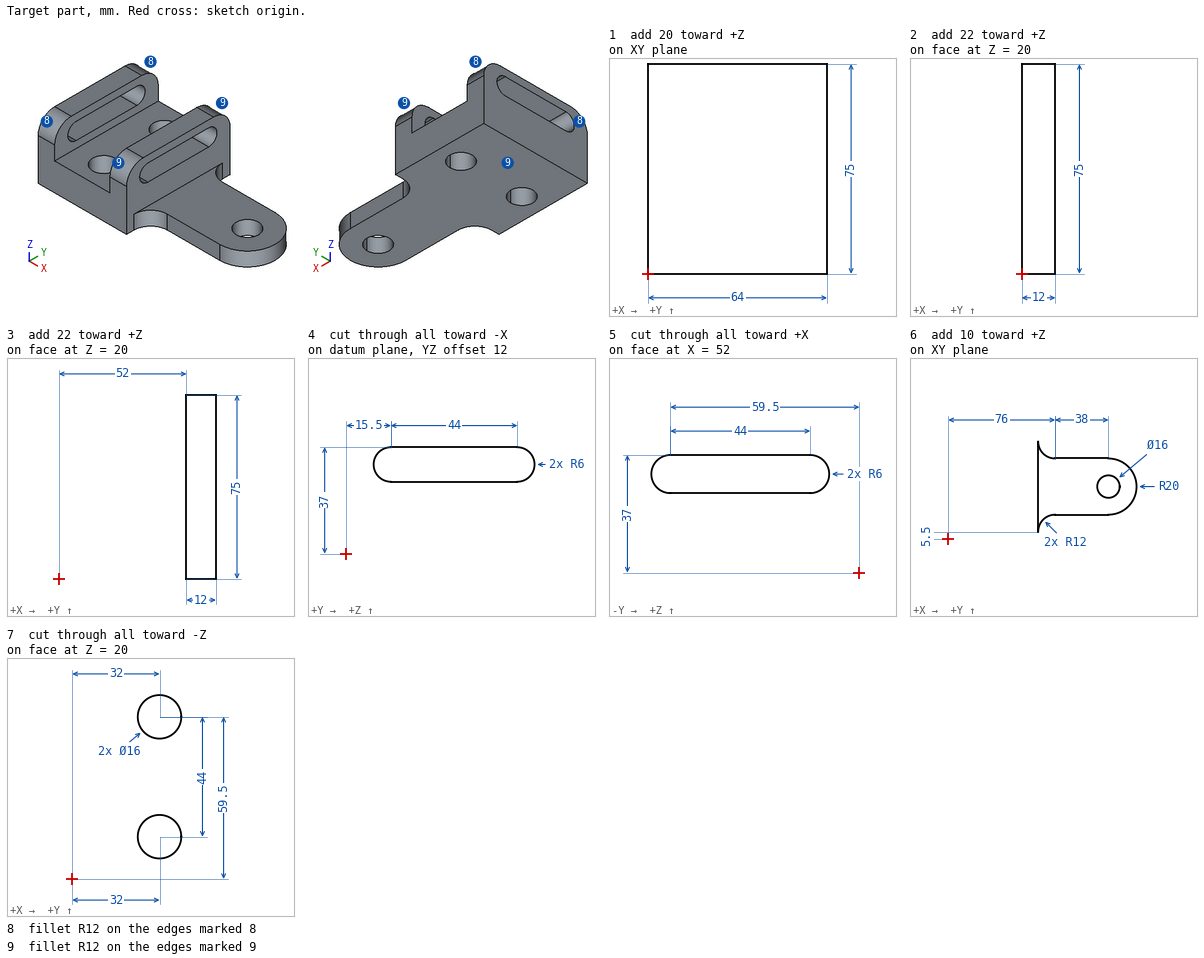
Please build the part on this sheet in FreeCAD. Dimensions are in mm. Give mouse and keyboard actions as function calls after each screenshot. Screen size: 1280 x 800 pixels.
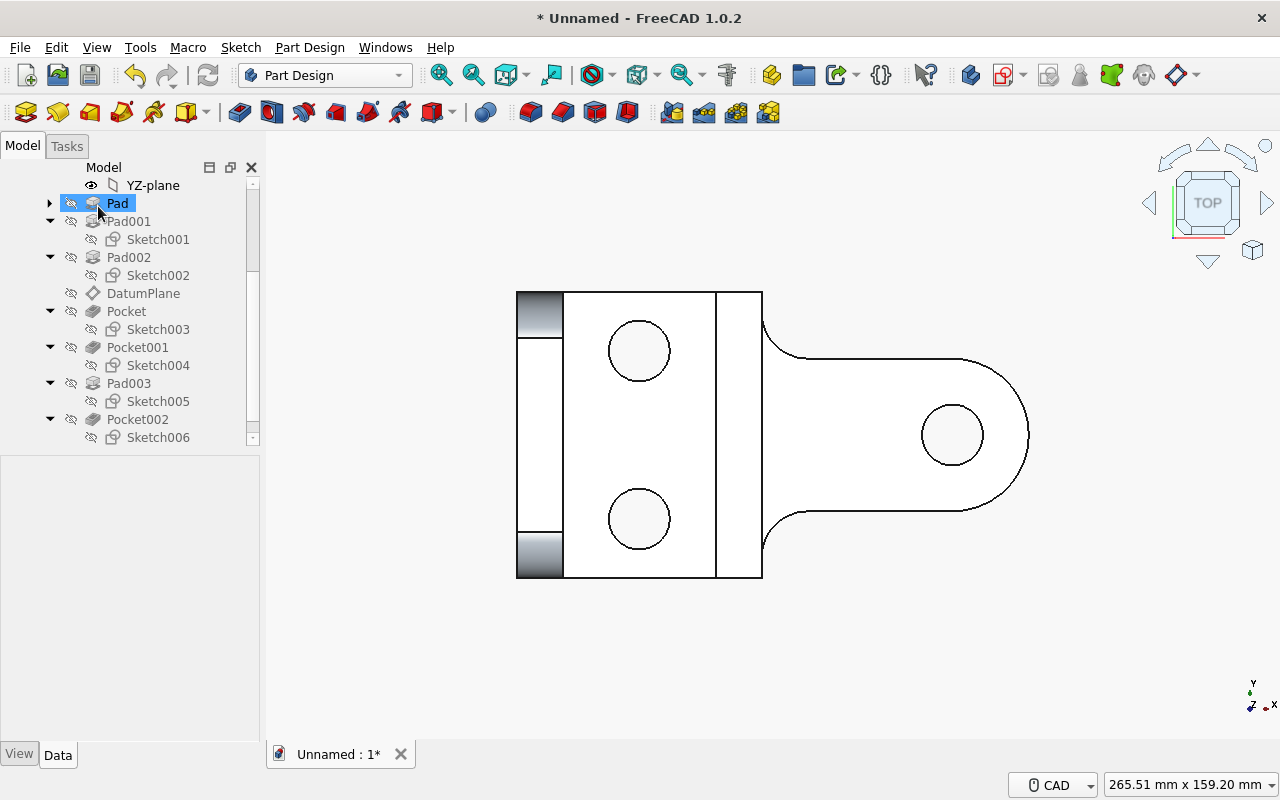
click(739, 577)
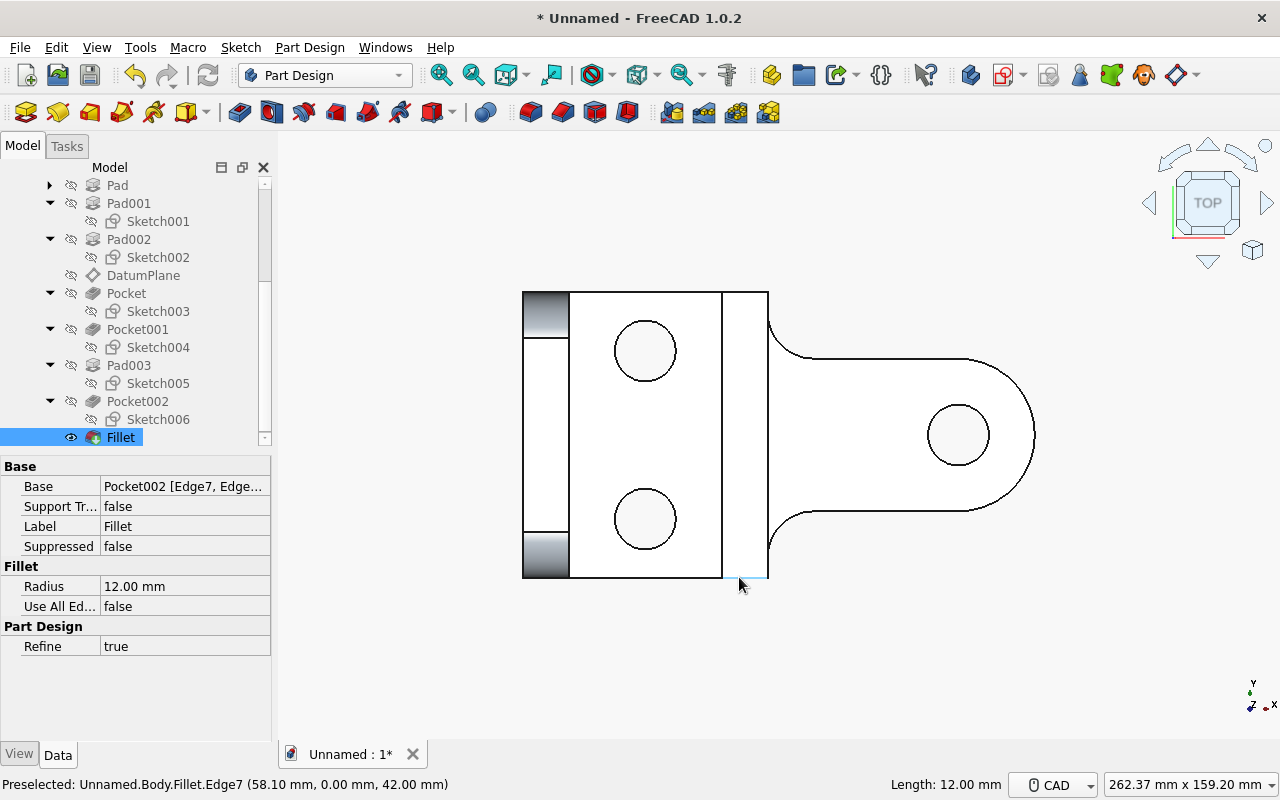
click(745, 291, ctrl)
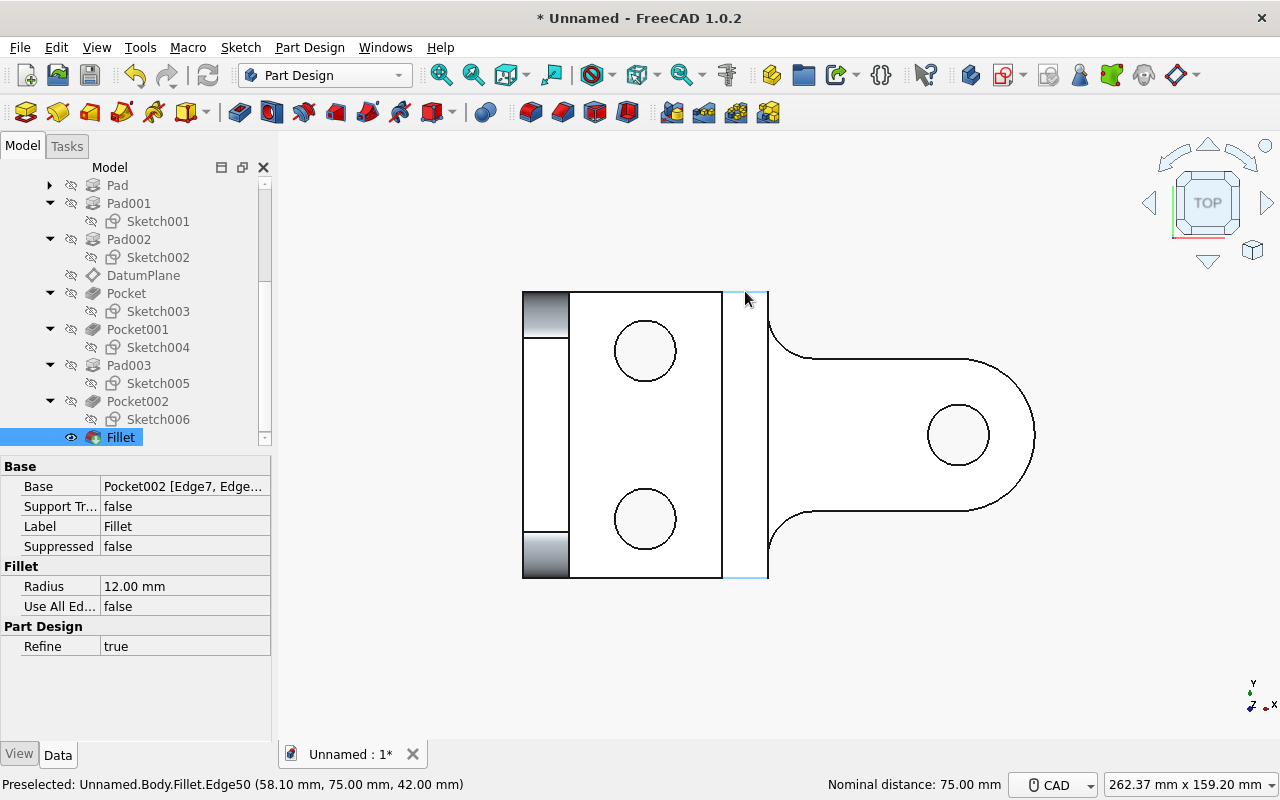
click(532, 112)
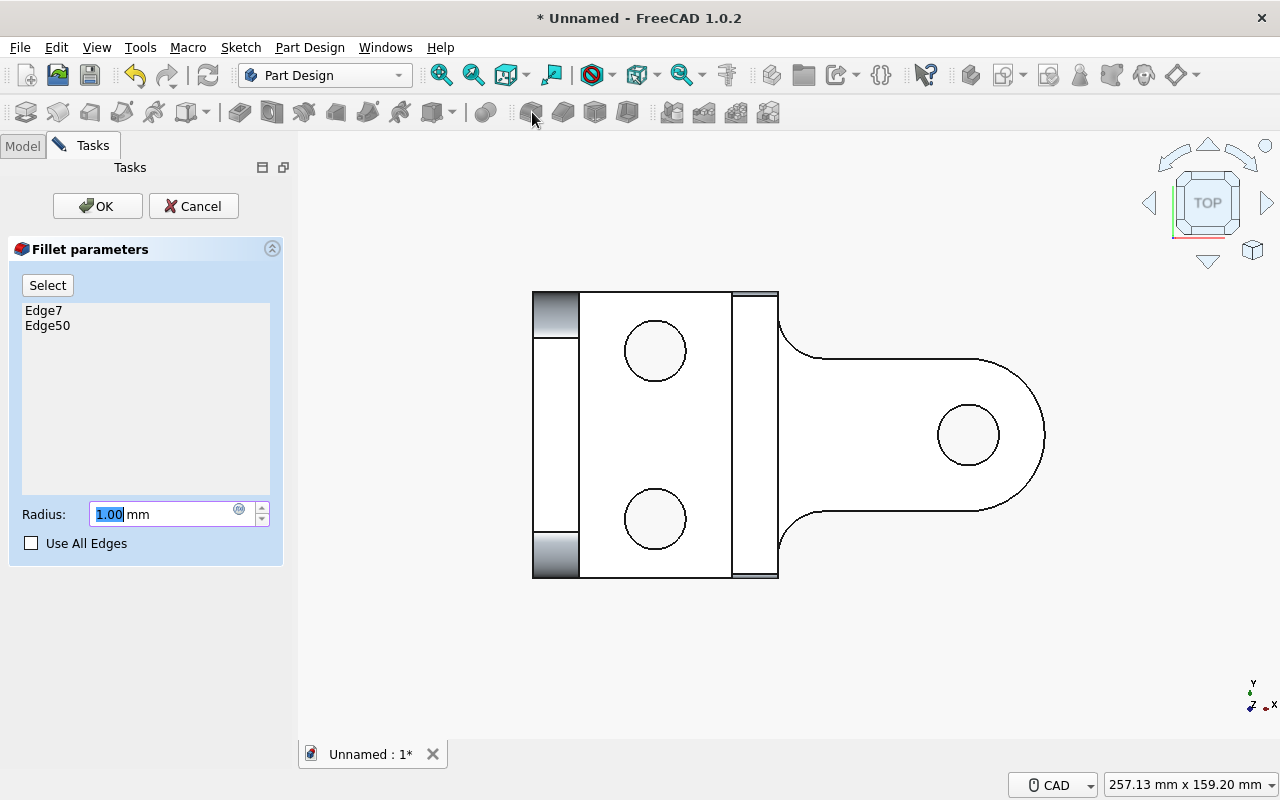
text(12)
key(Tab)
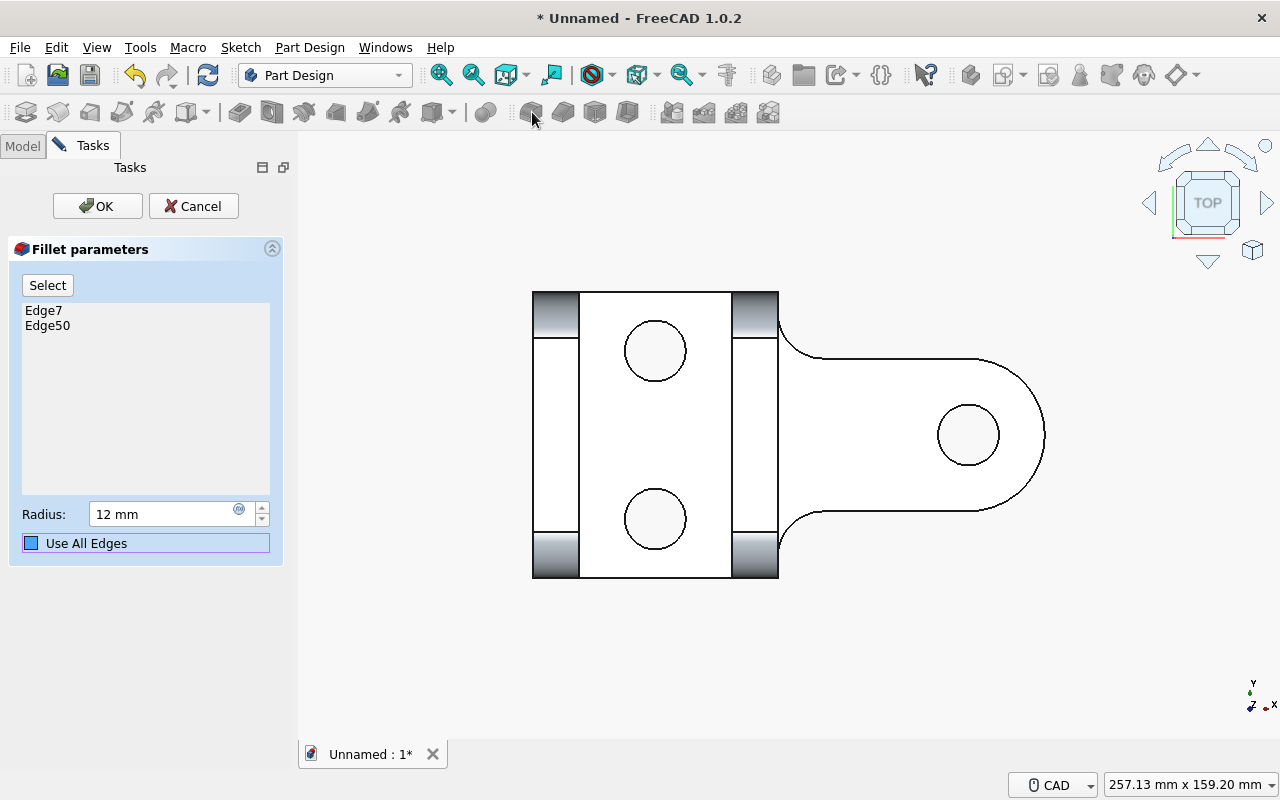
click(98, 206)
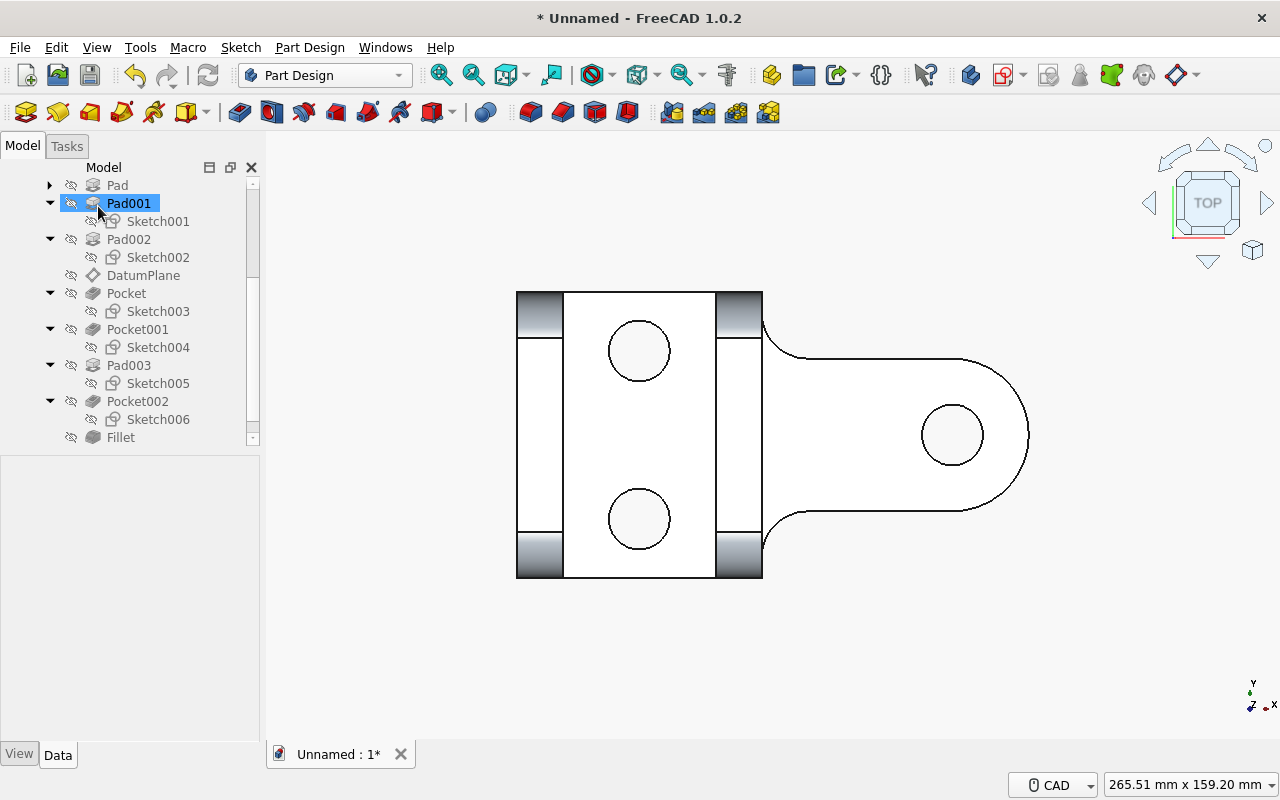
key(0)